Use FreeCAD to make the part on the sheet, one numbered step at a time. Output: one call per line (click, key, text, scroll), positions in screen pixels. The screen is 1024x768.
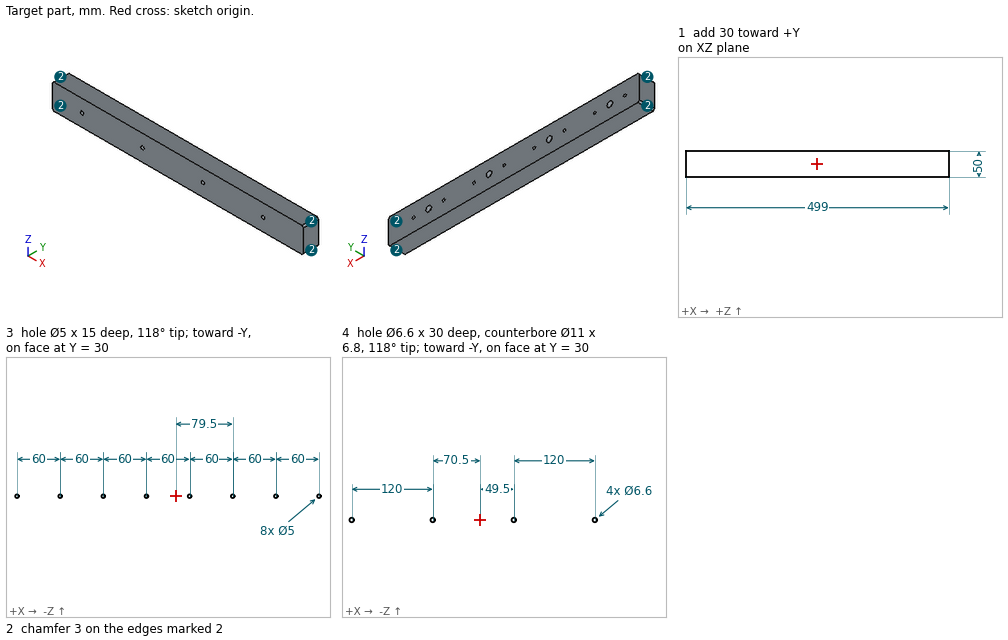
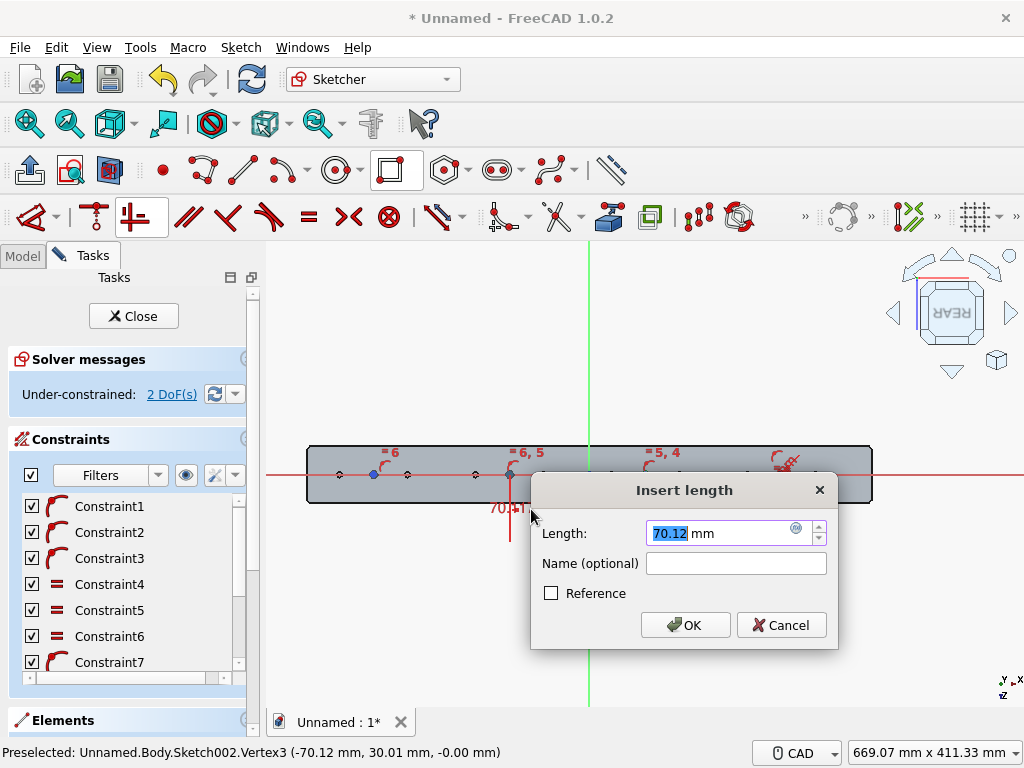
text(70.5)
key(Return)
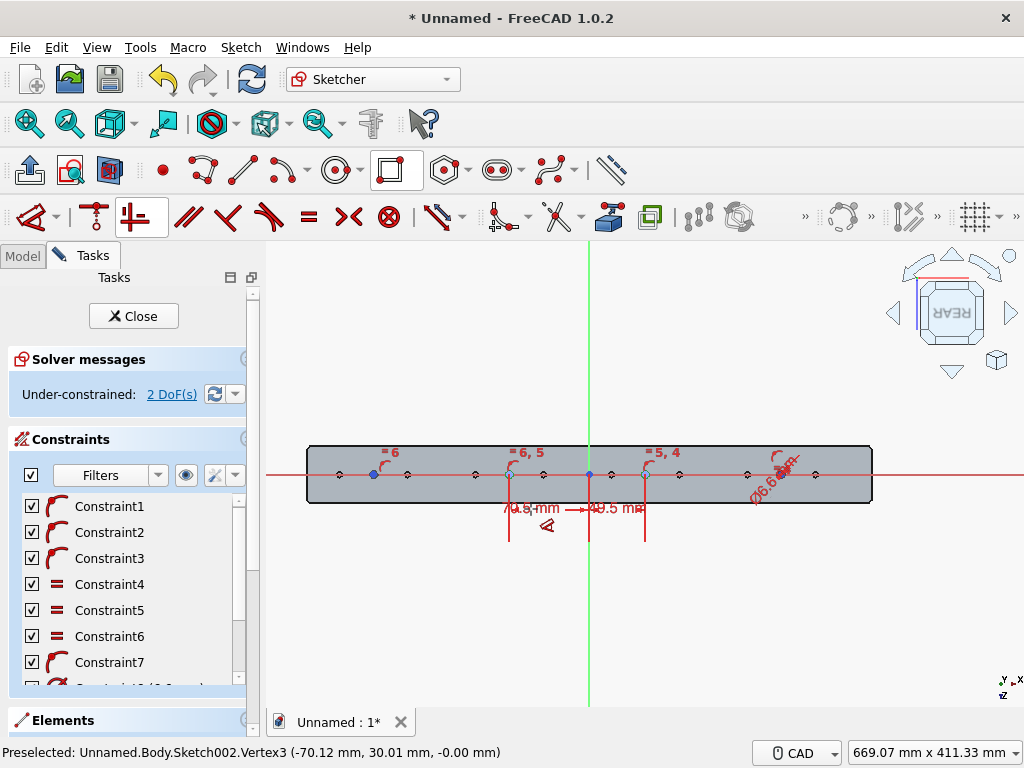
click(781, 475)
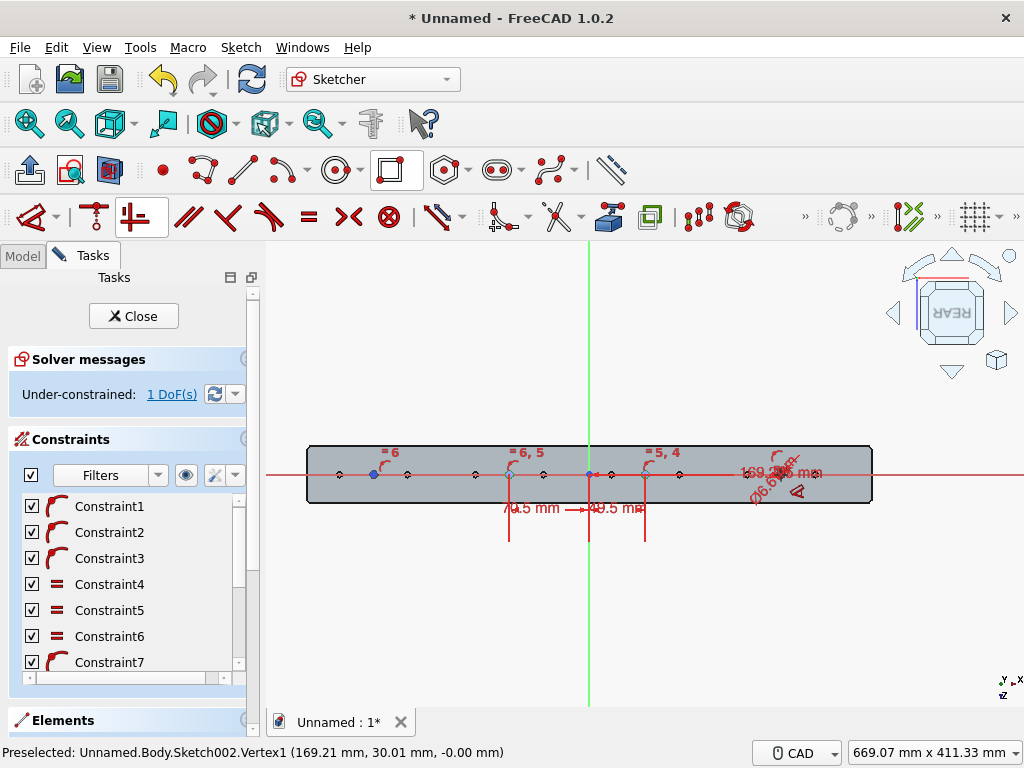
click(645, 475)
click(713, 509)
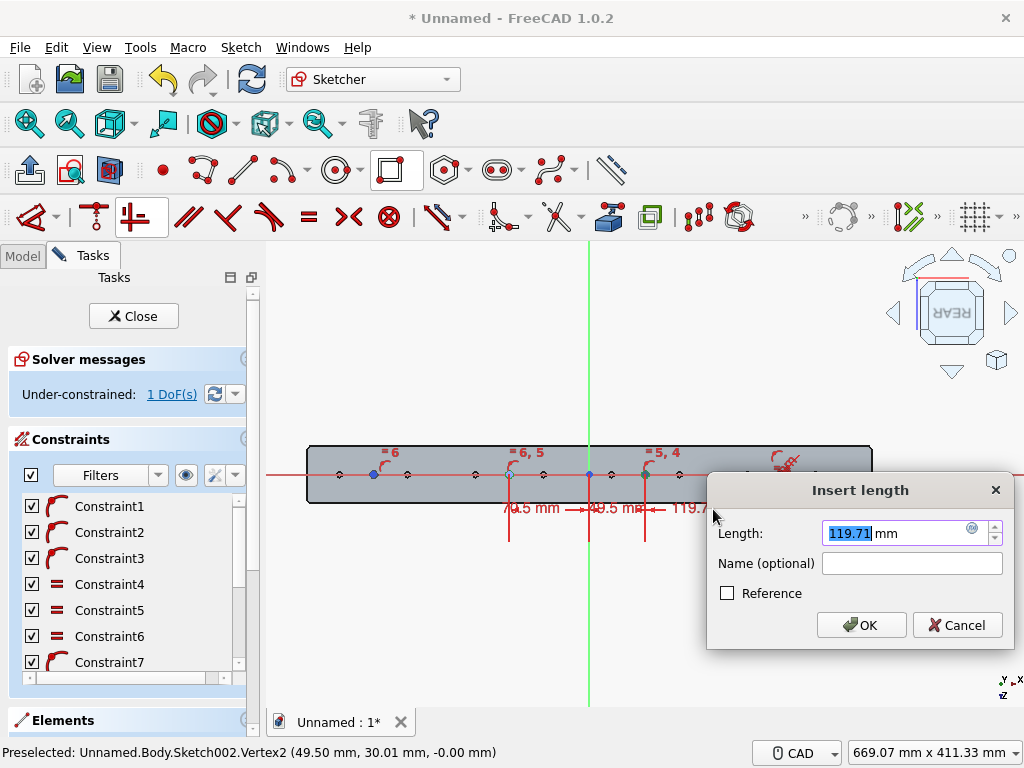
text(120)
key(Return)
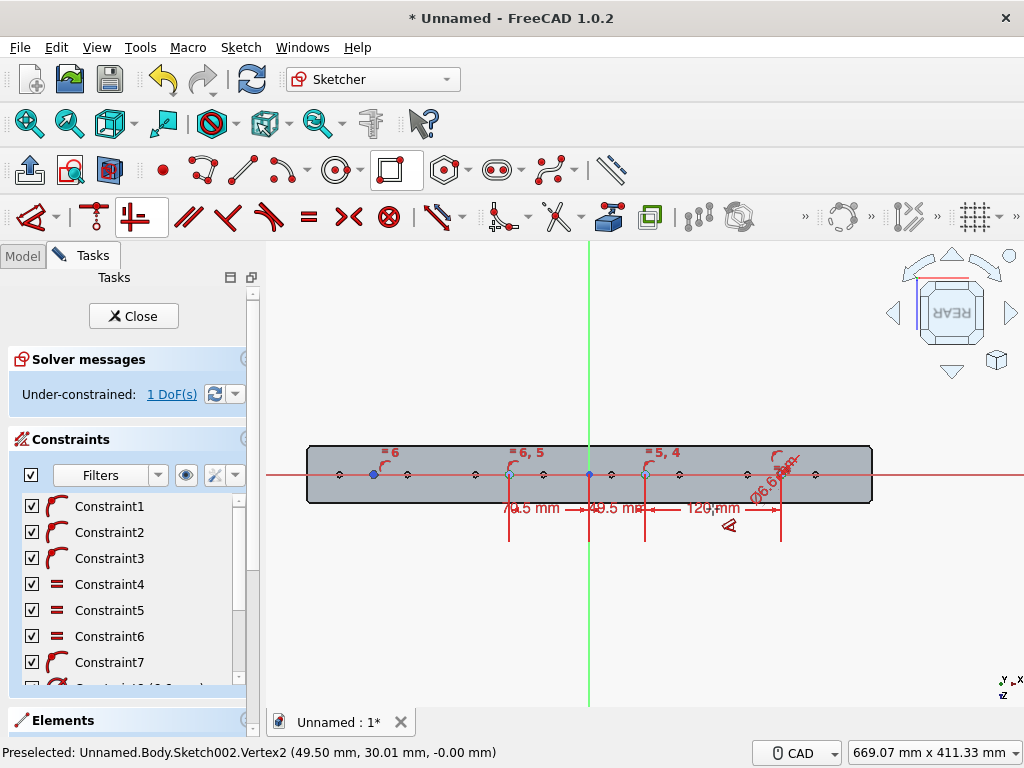
click(509, 475)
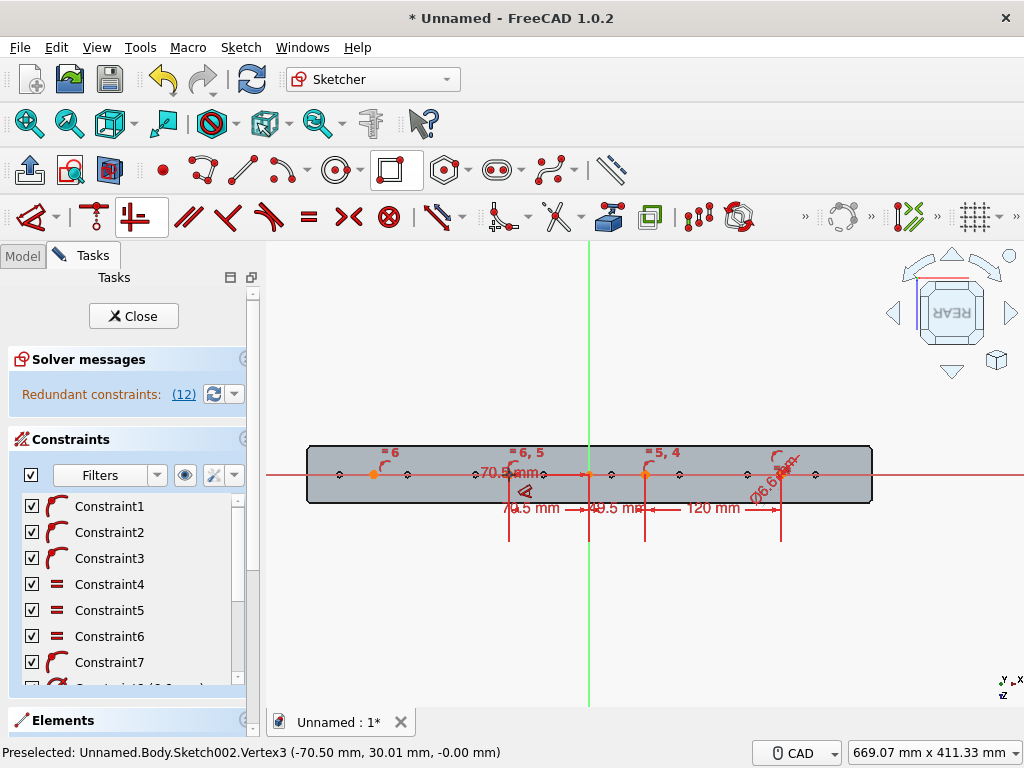
click(374, 475)
click(442, 509)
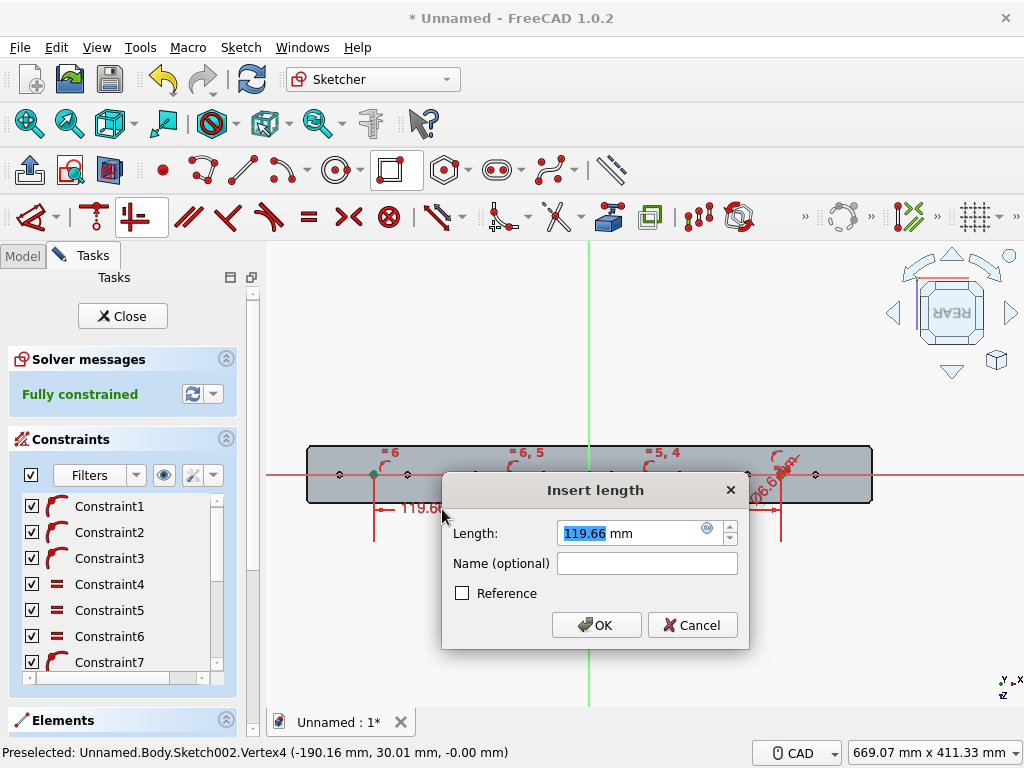
text(120)
key(Return)
key(Escape)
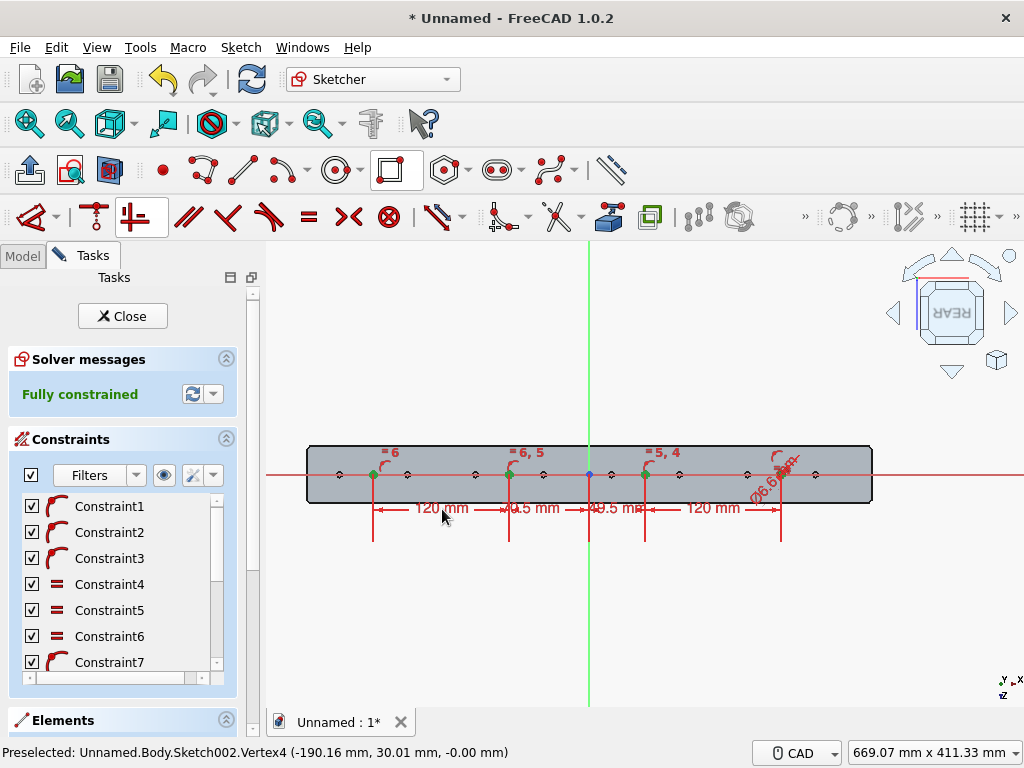
click(123, 316)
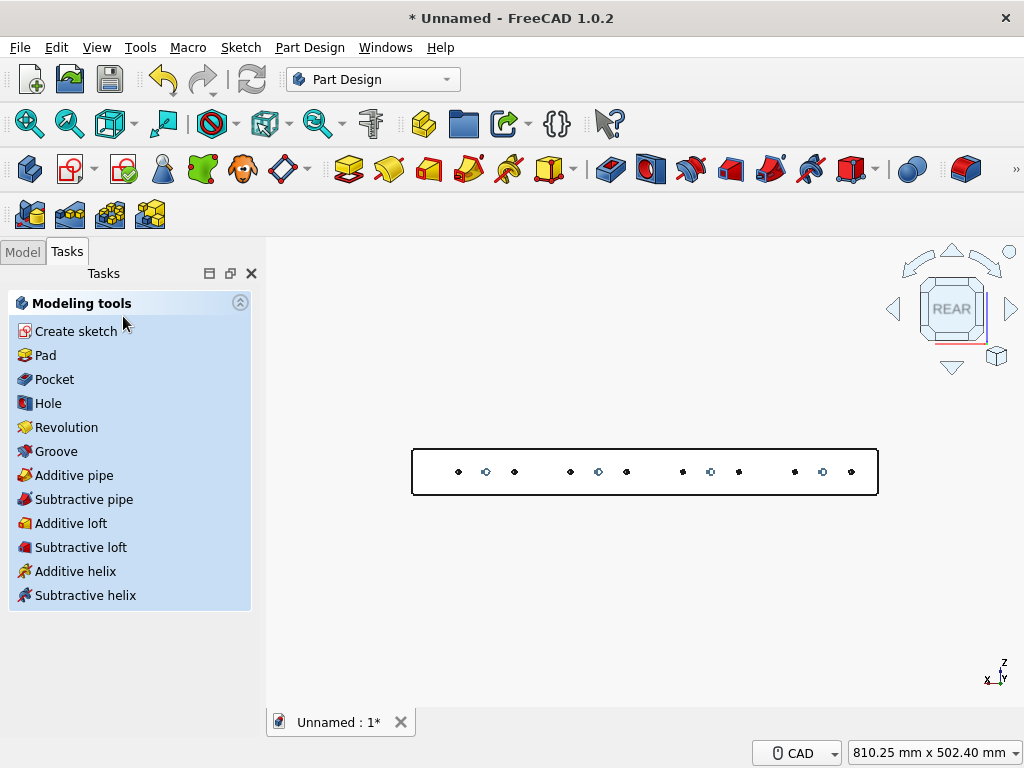
click(652, 170)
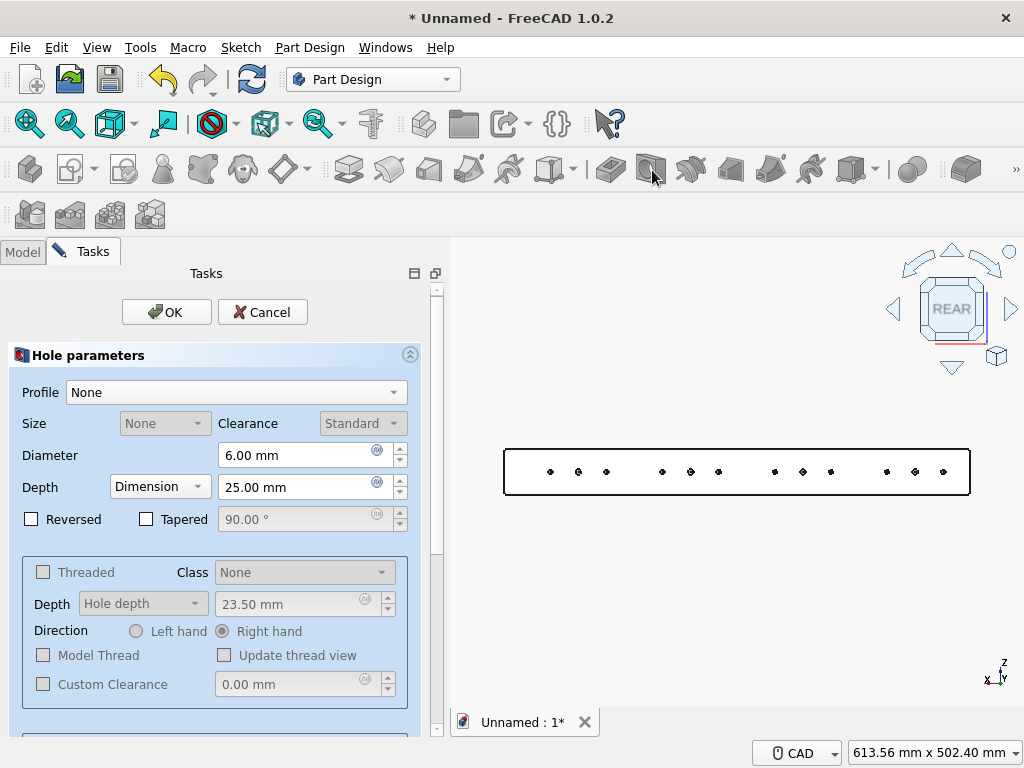
triple_click(305, 455)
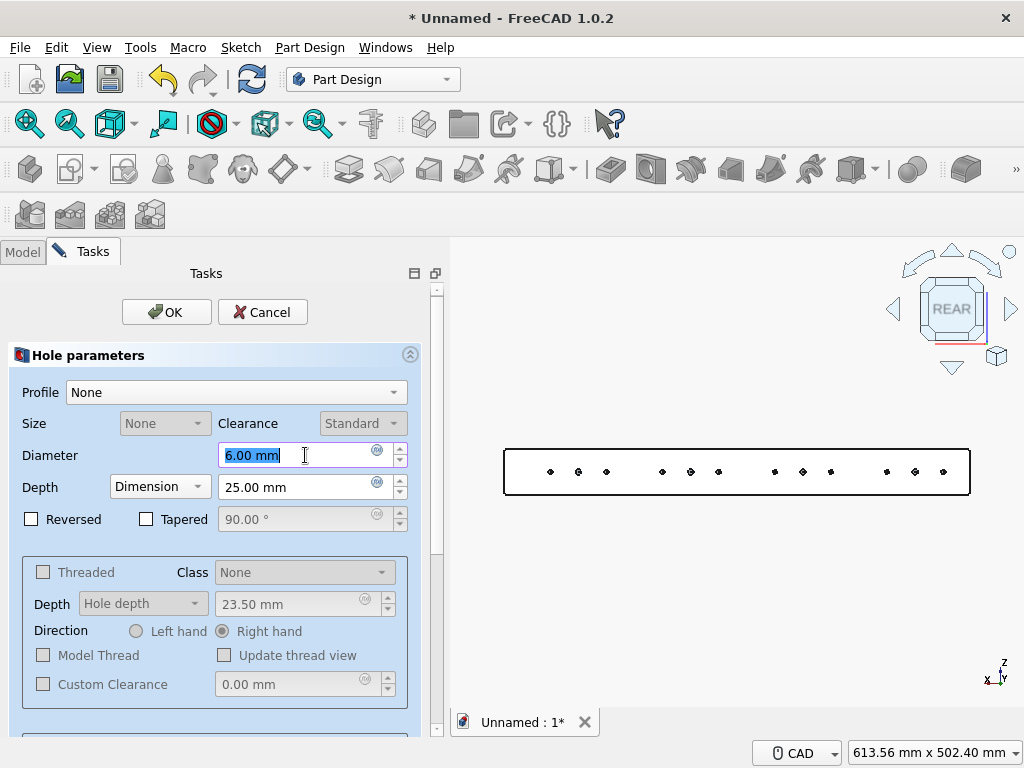
text(6.6)
key(Tab)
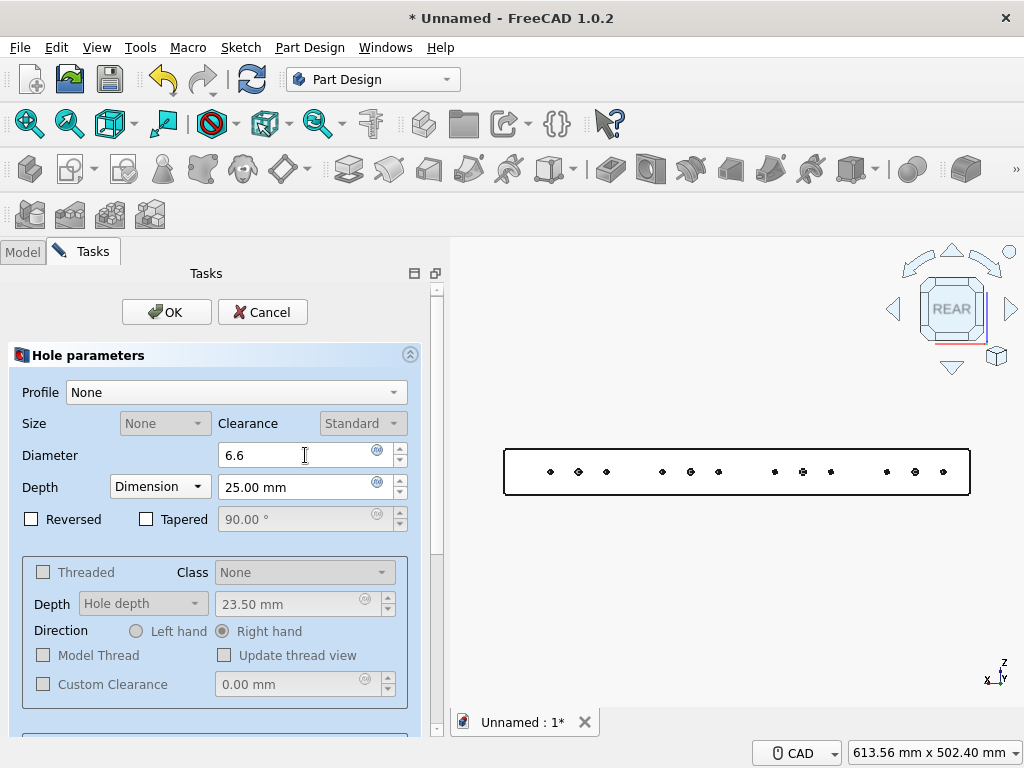
triple_click(305, 487)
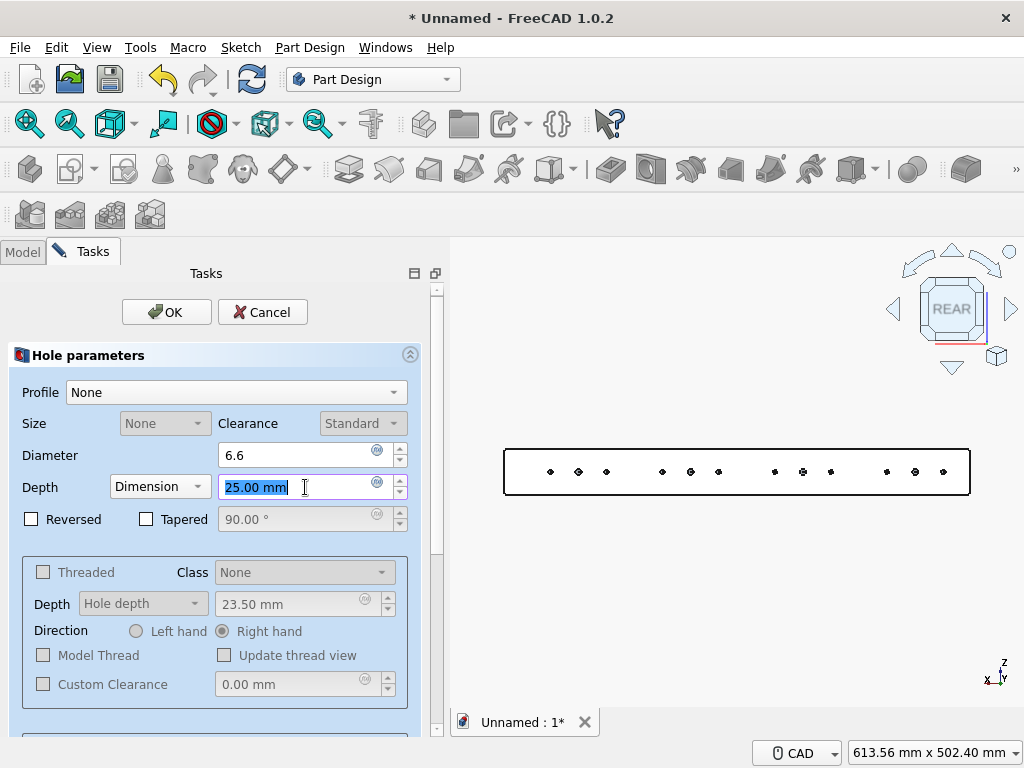
text(30)
key(Tab)